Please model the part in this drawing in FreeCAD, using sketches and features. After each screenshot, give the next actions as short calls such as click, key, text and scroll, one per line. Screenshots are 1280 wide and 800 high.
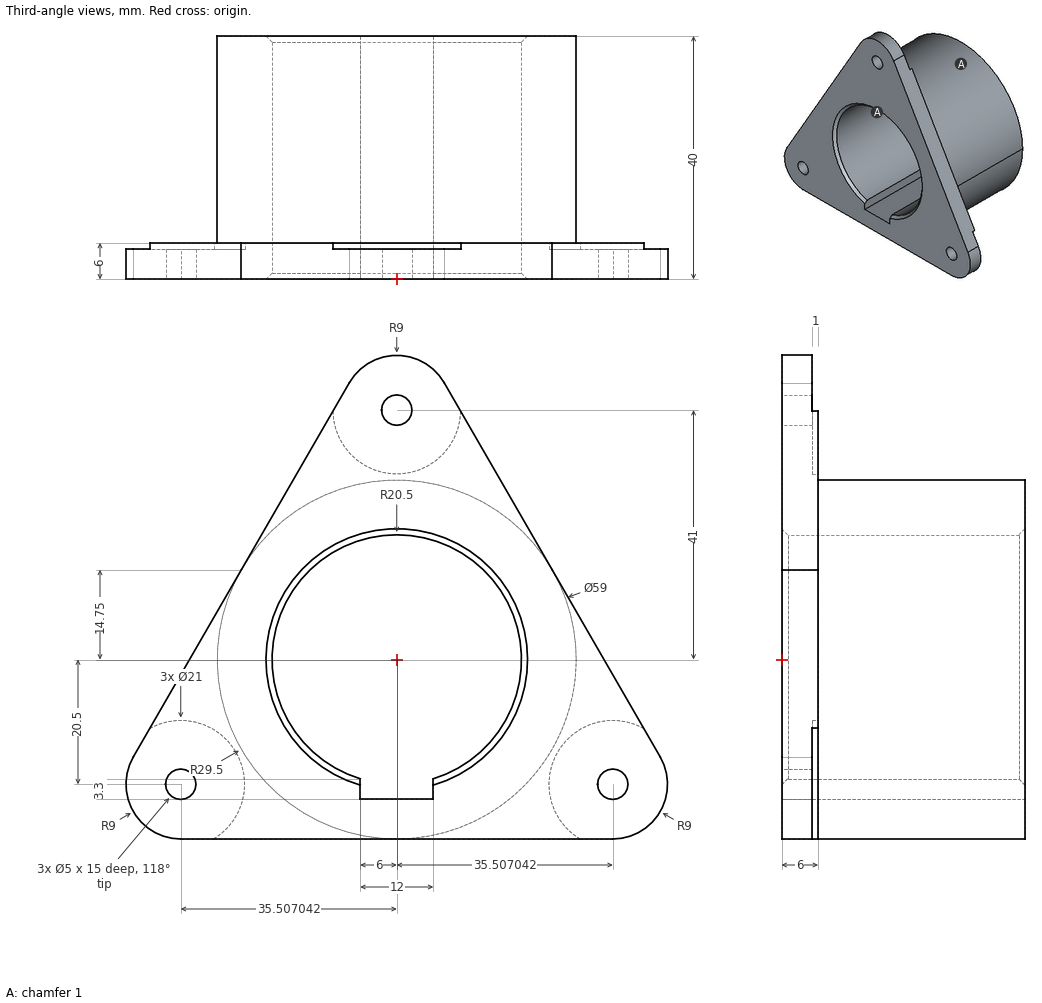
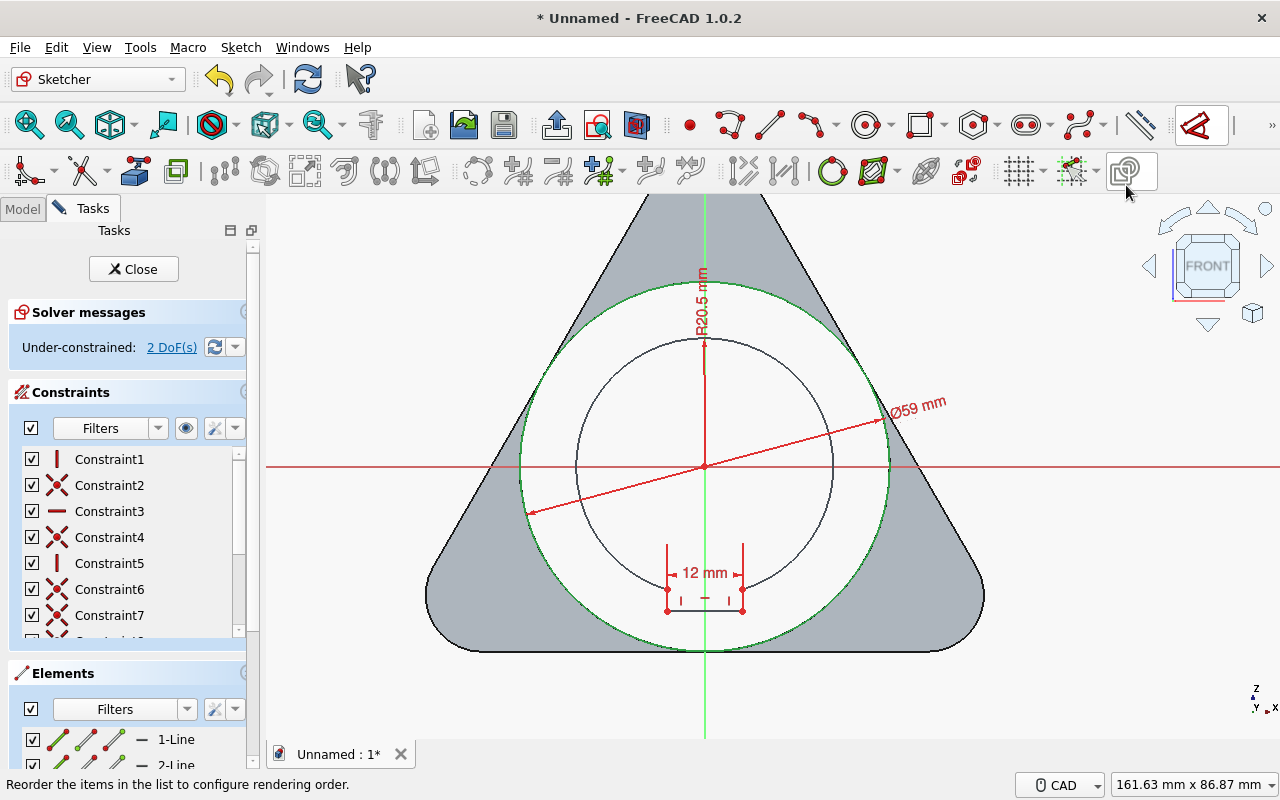
click(667, 590)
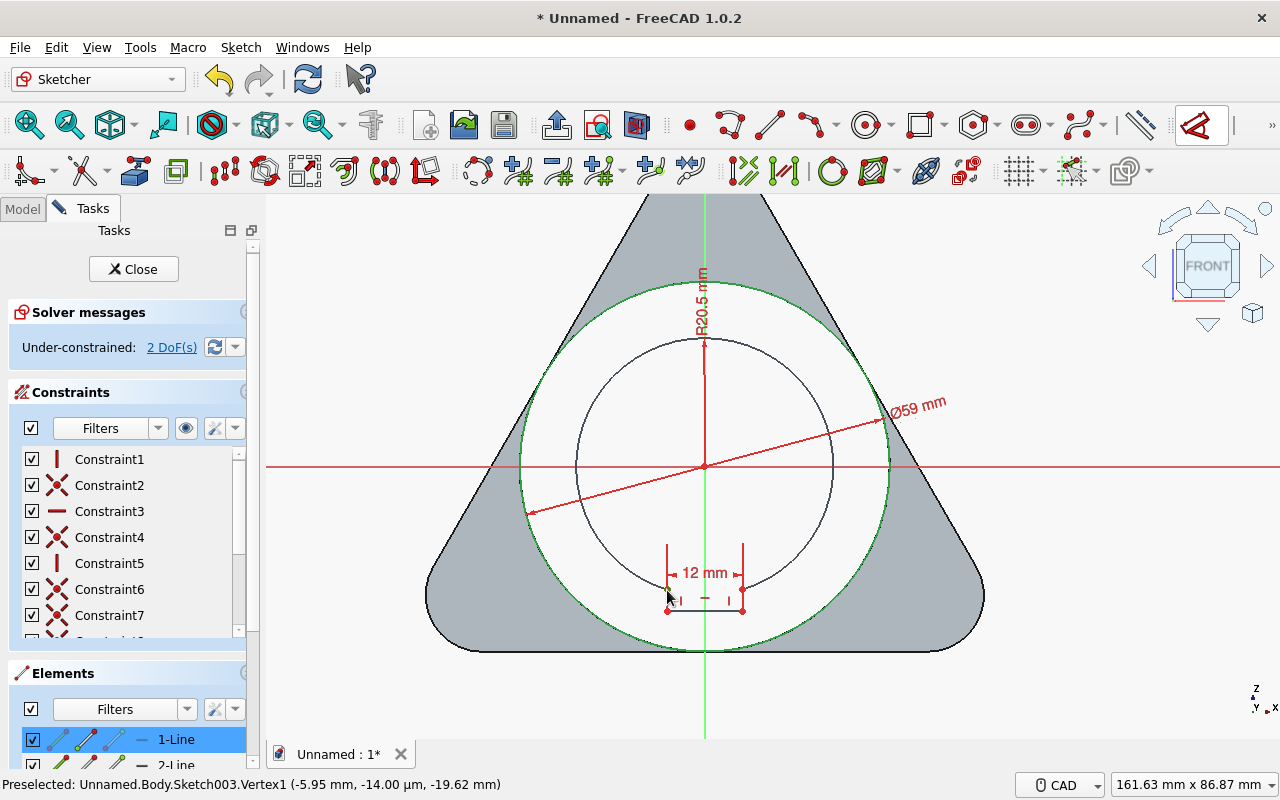
click(1222, 126)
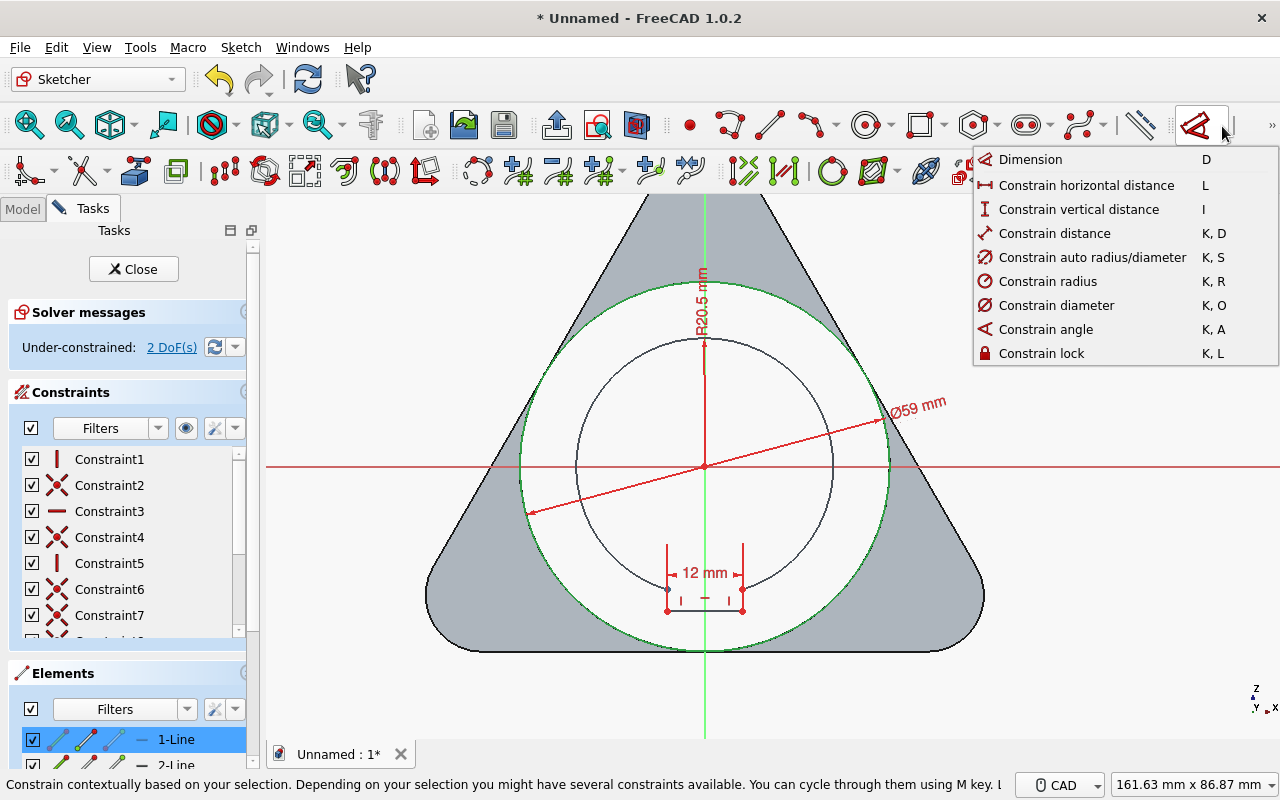
click(1126, 185)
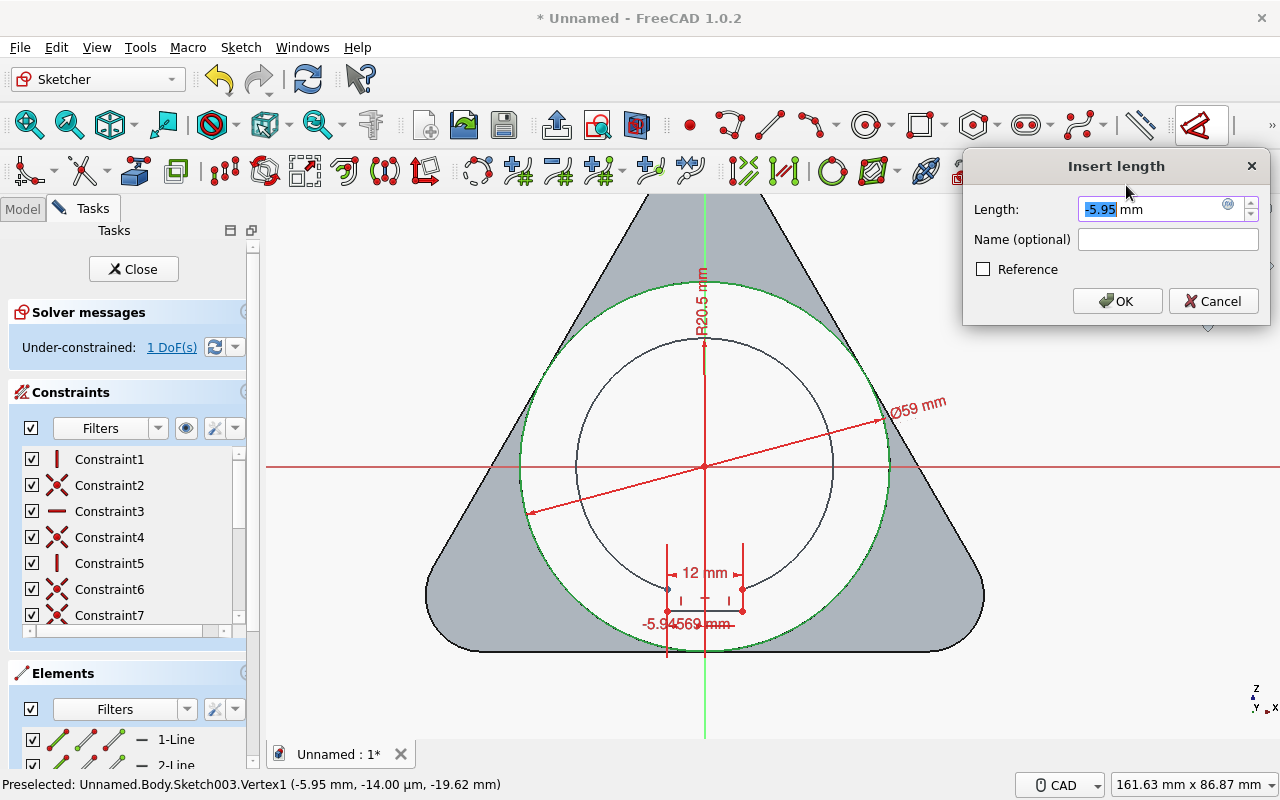
text(-6)
key(Return)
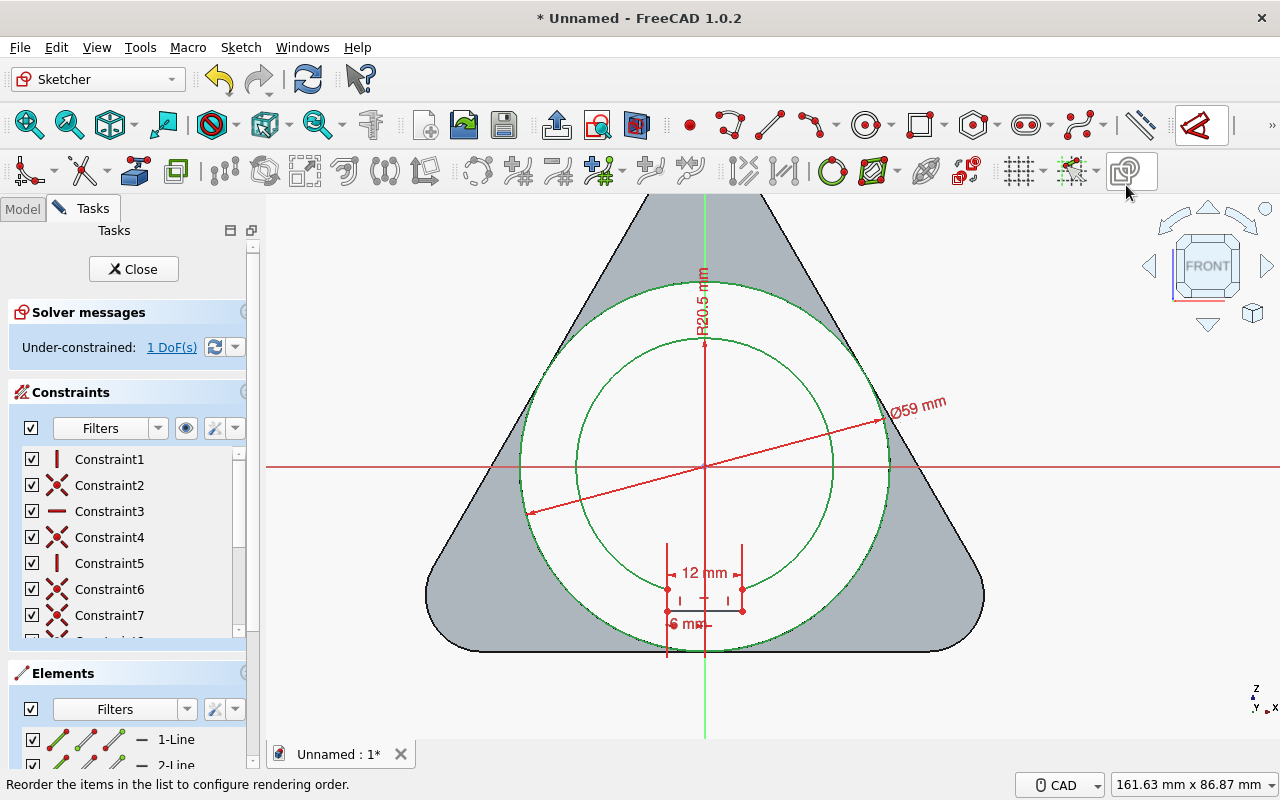
scroll(667, 601, up, 4)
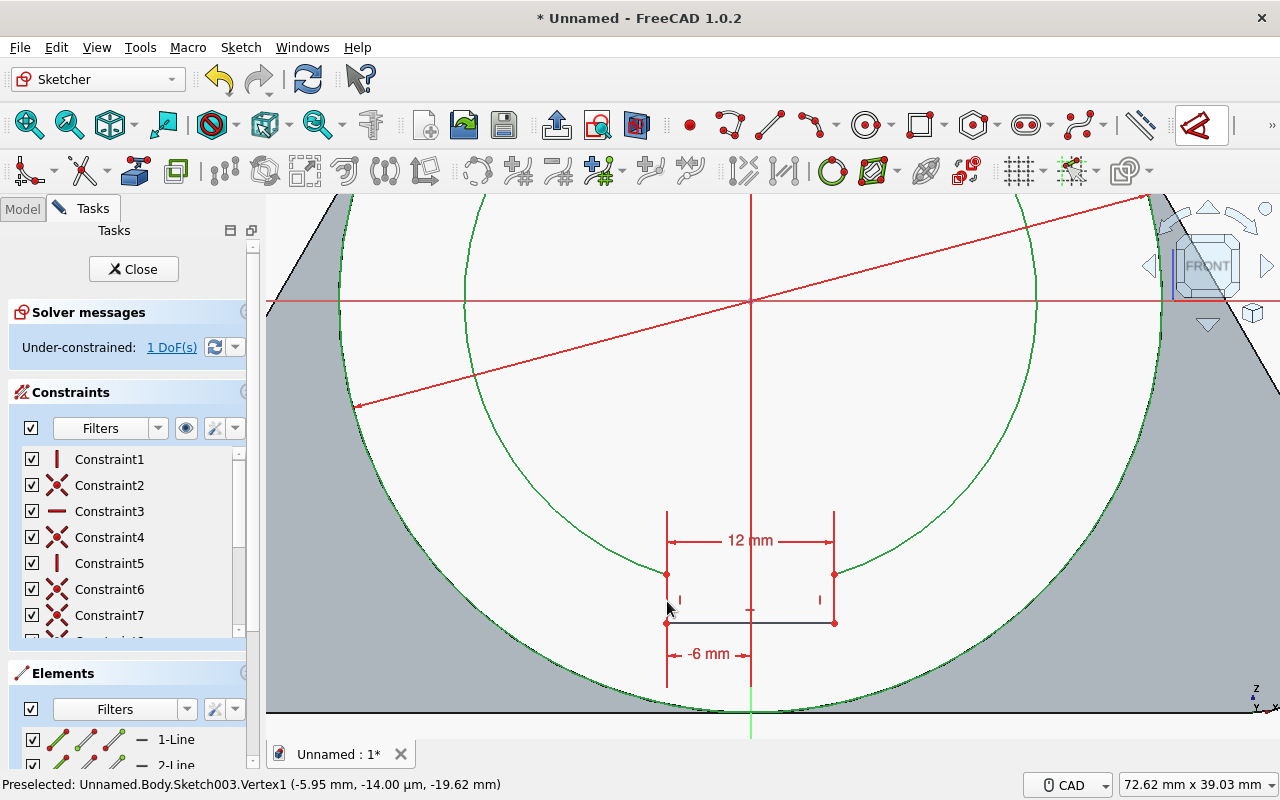
click(667, 599)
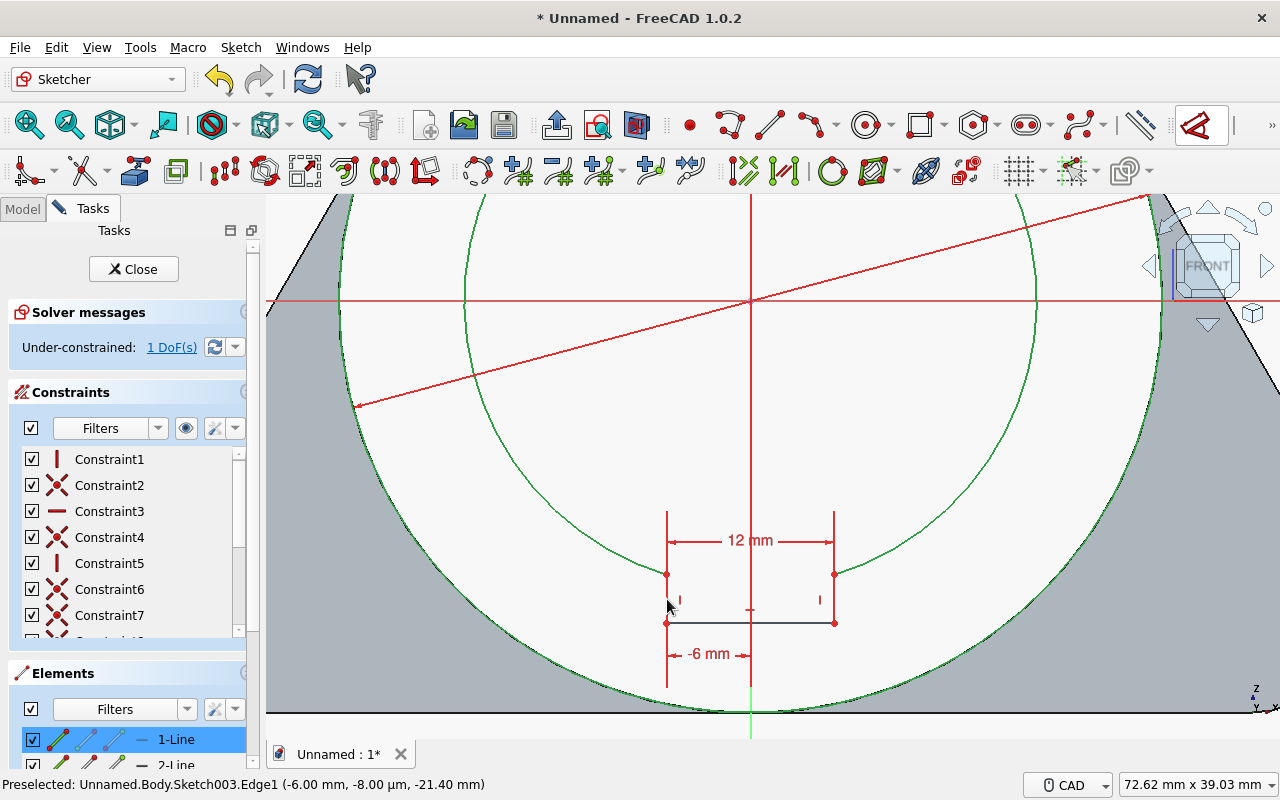
key(i)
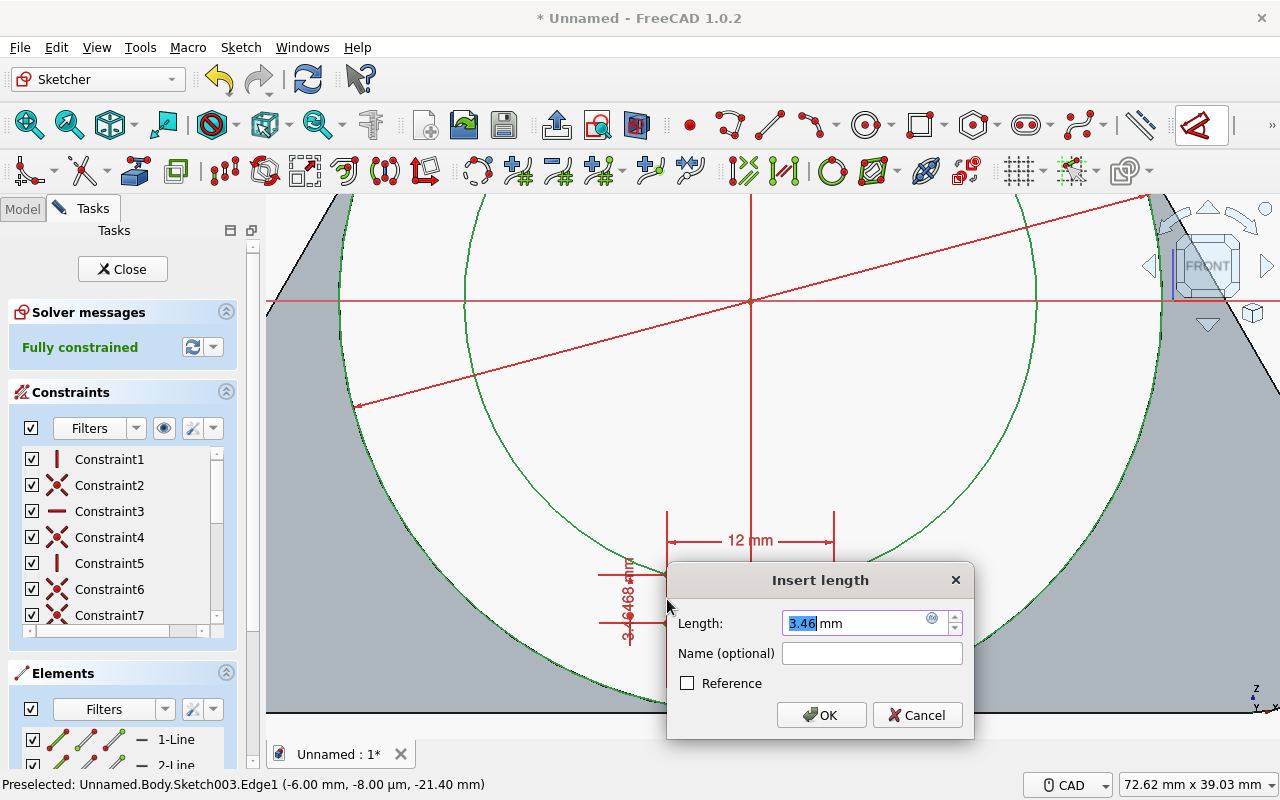
text(3.3)
key(Return)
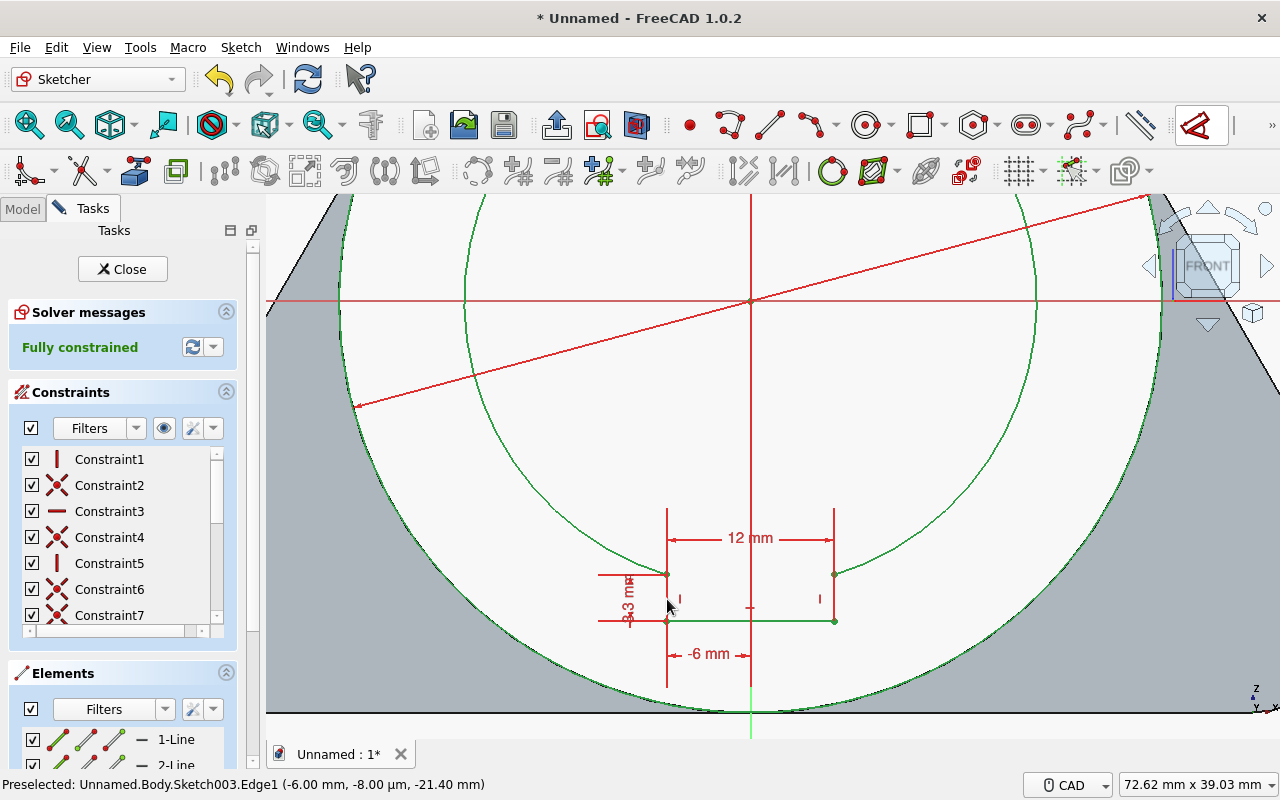
click(123, 269)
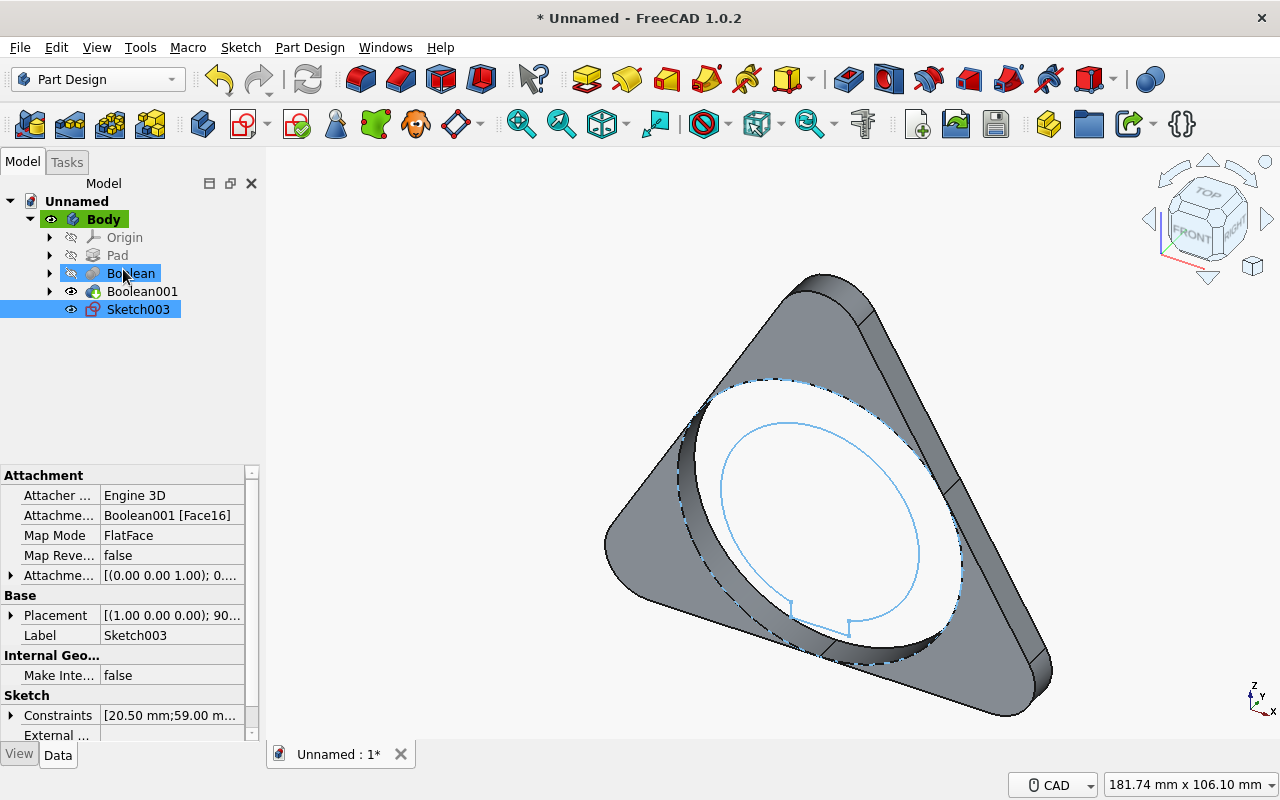
click(588, 80)